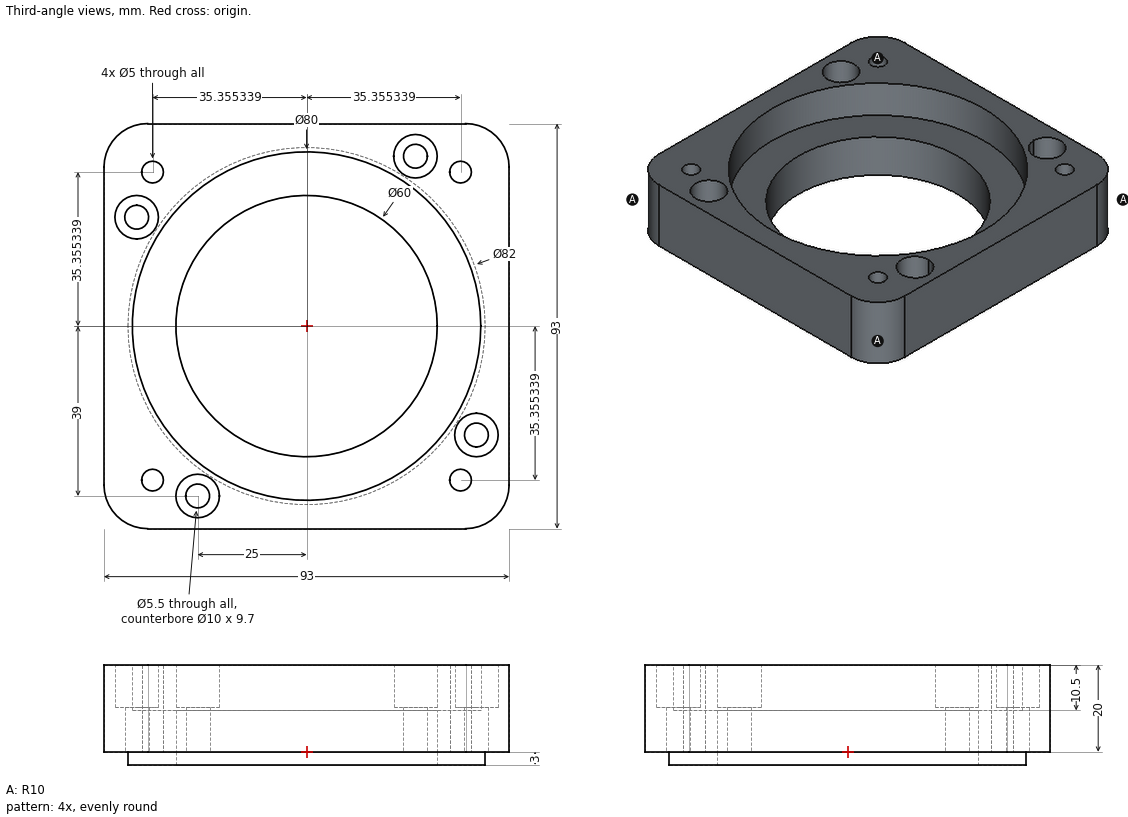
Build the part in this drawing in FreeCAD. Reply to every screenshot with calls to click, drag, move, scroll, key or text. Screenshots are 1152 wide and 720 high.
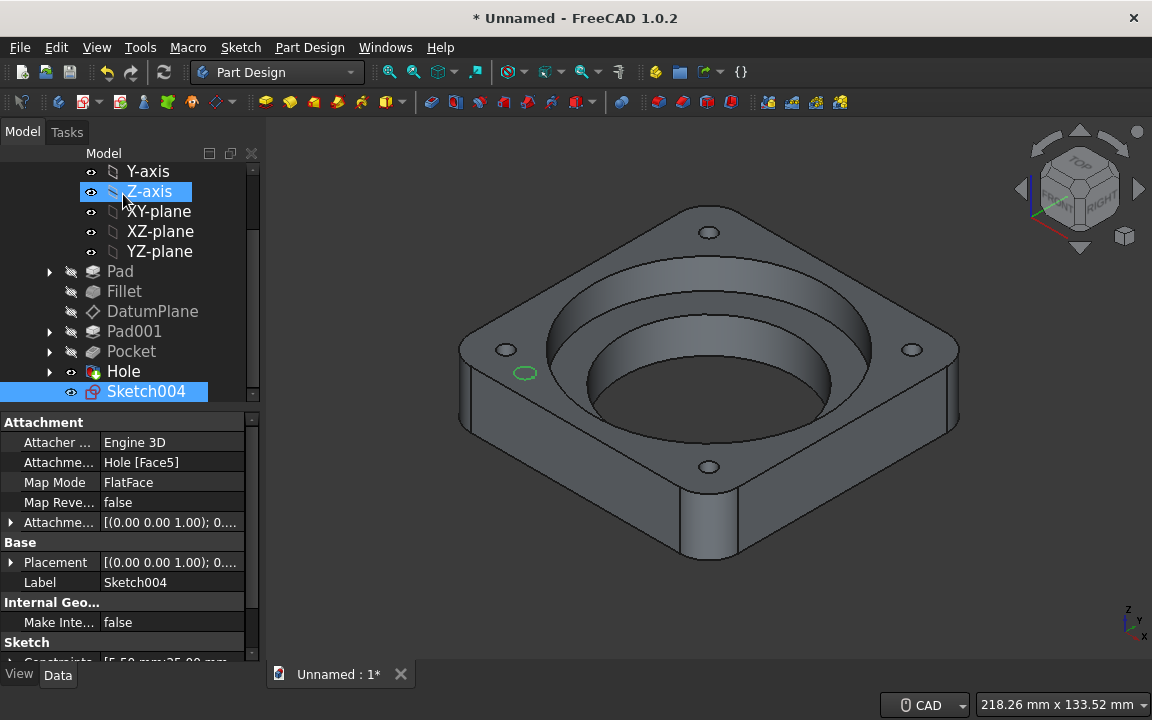
click(456, 102)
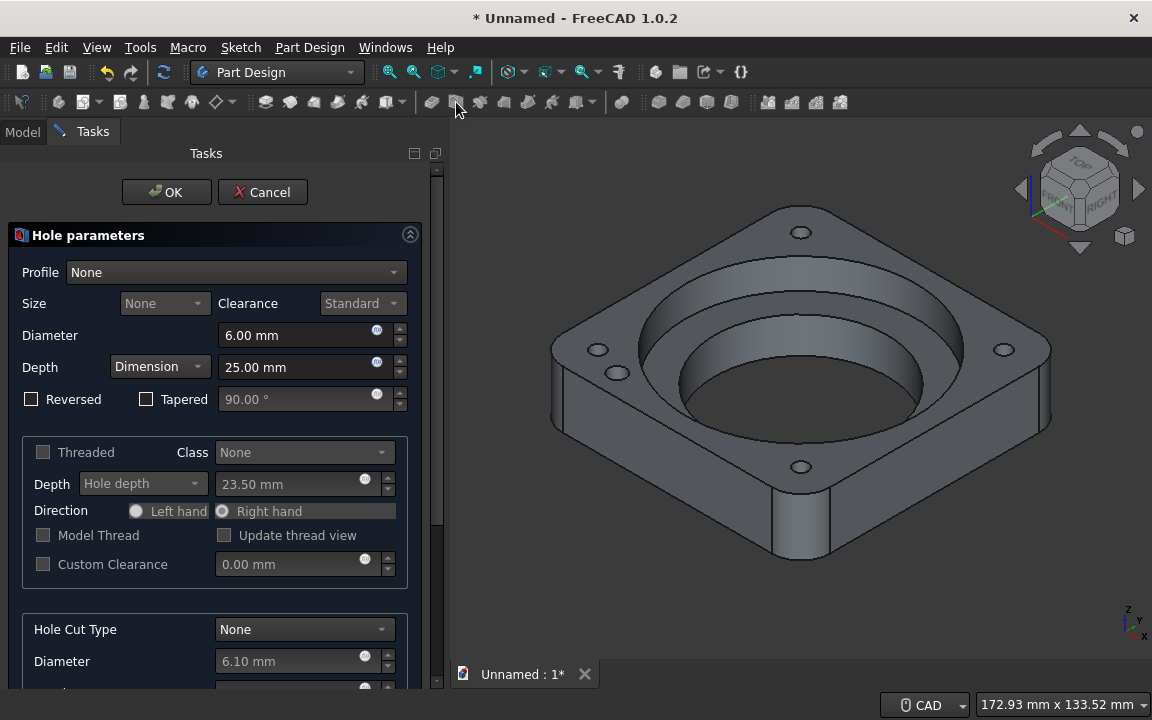
triple_click(305, 335)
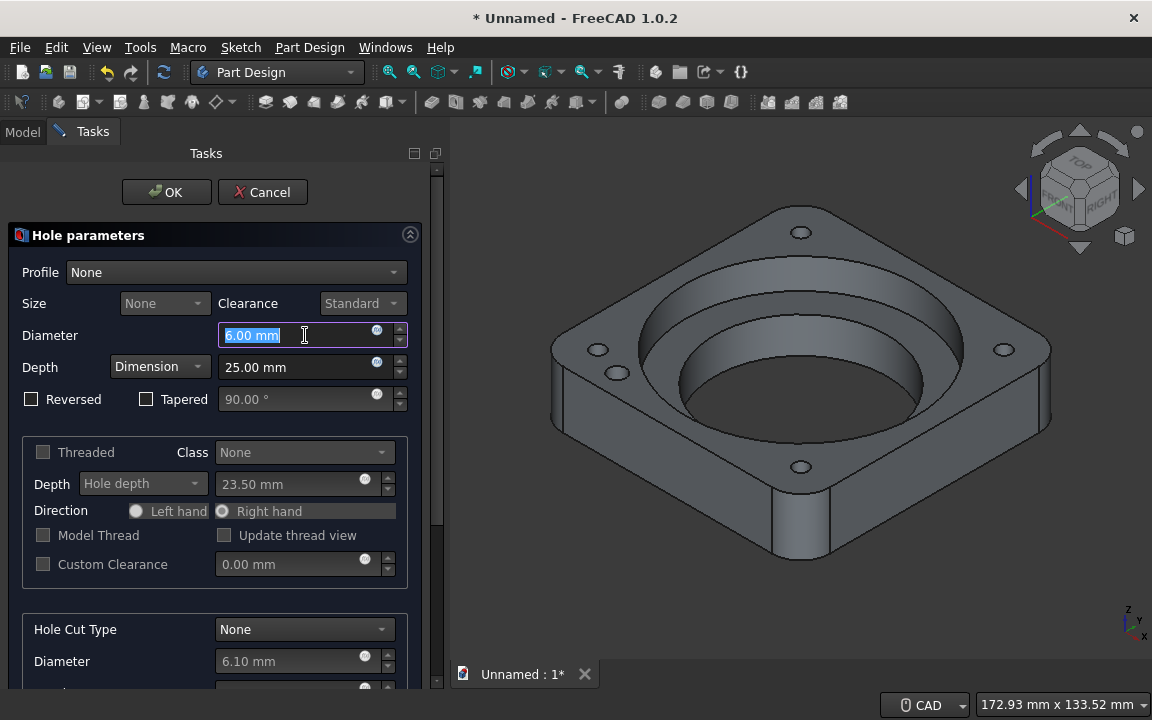
text(5.5)
key(Tab)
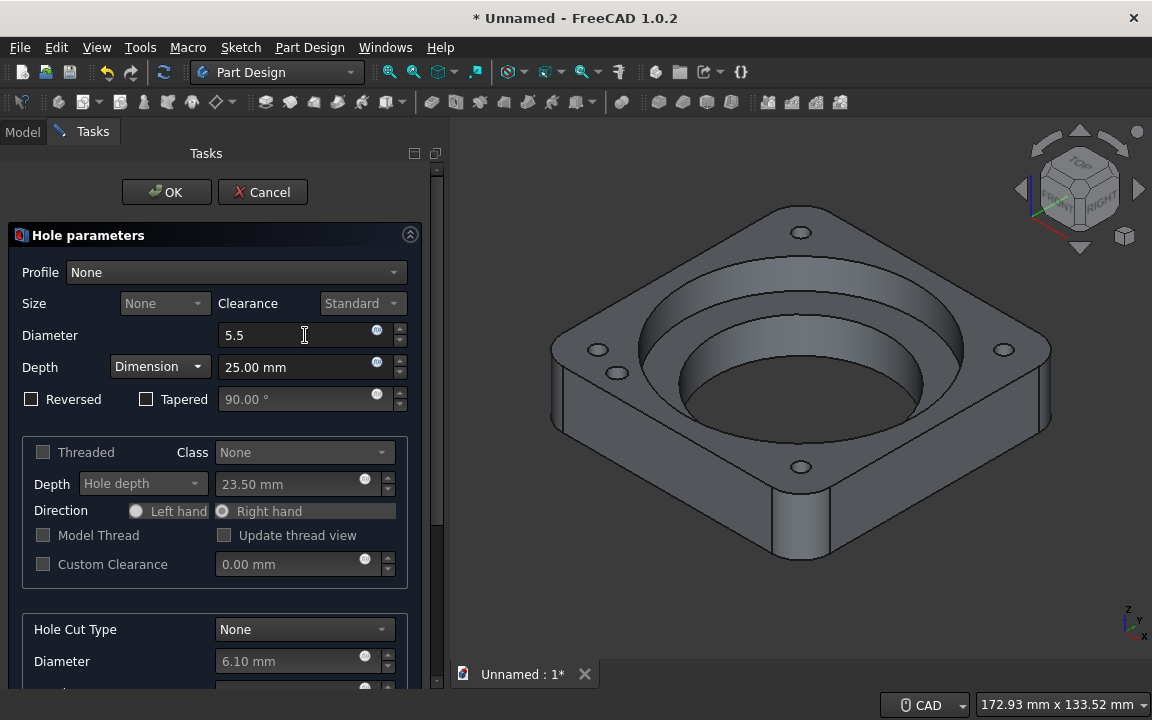
click(161, 366)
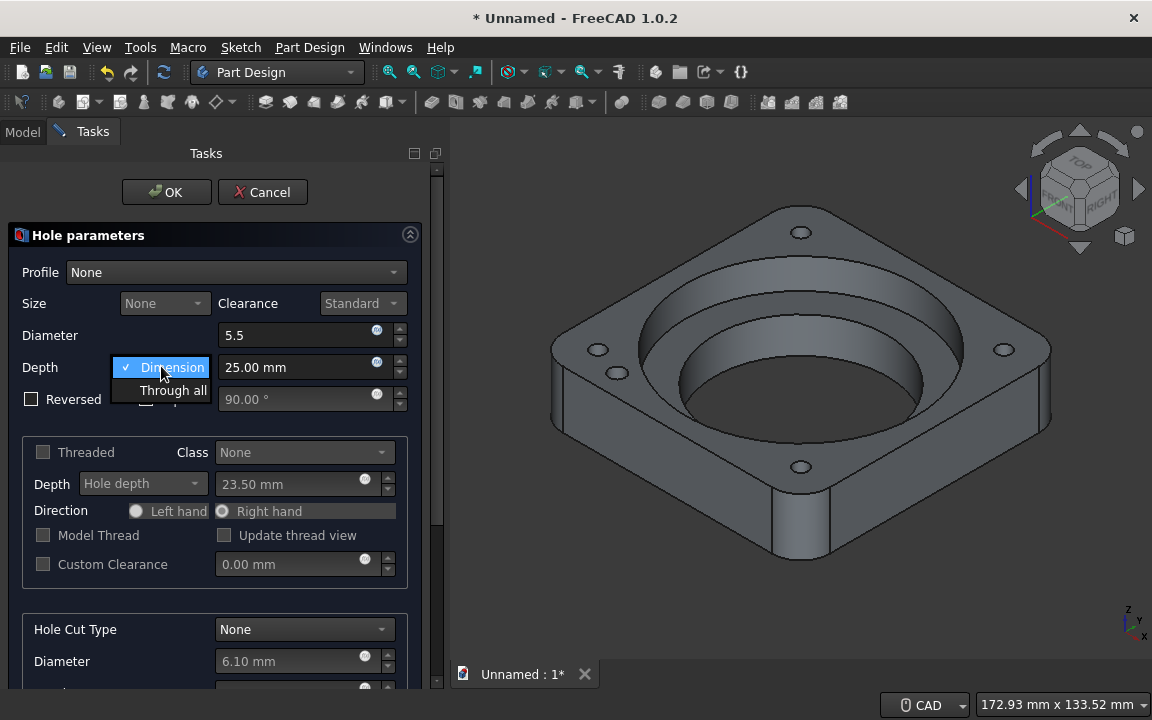
click(160, 390)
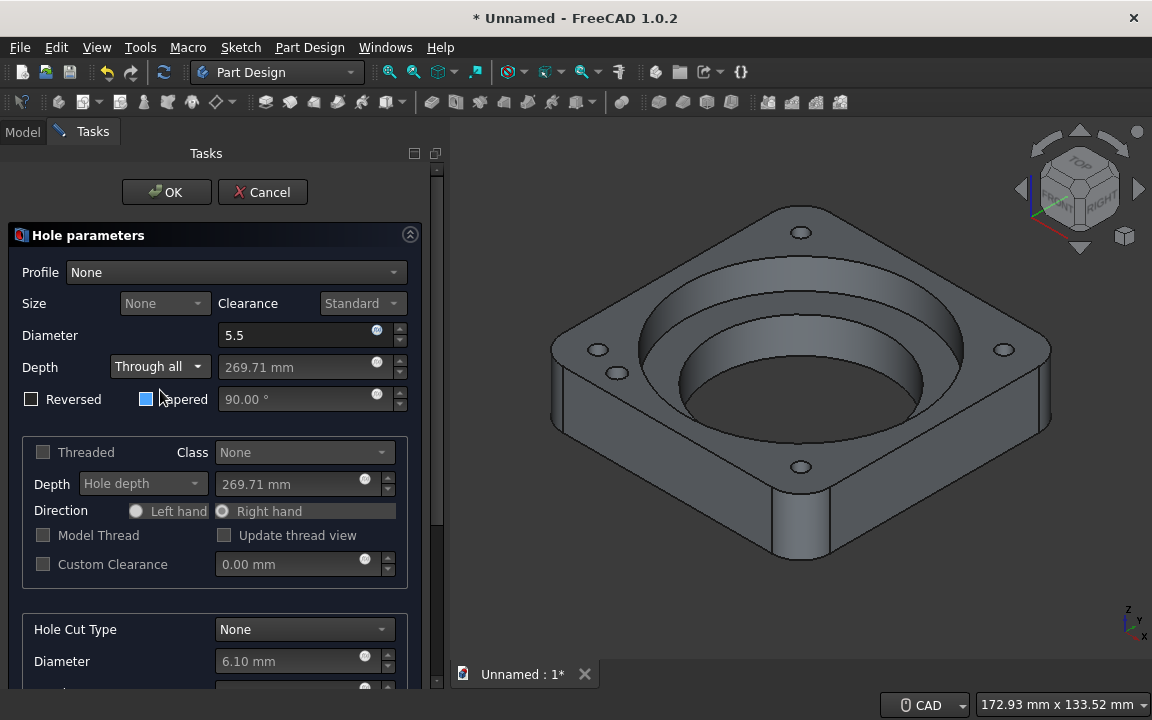
click(306, 630)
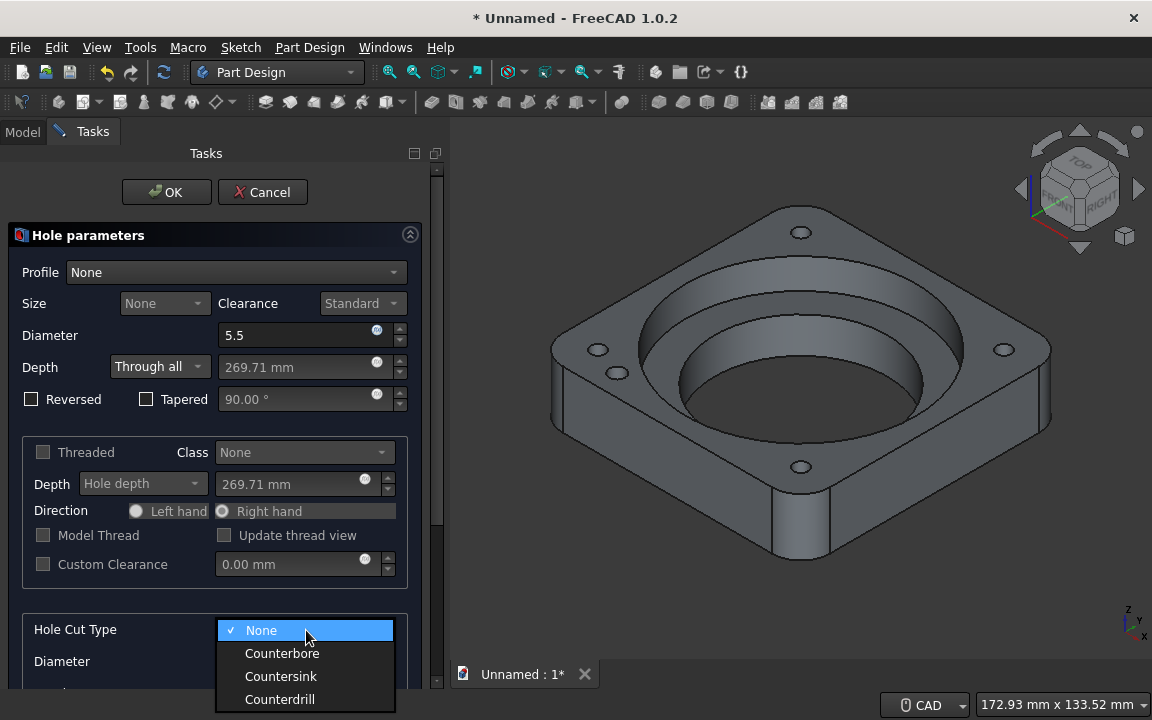
click(304, 654)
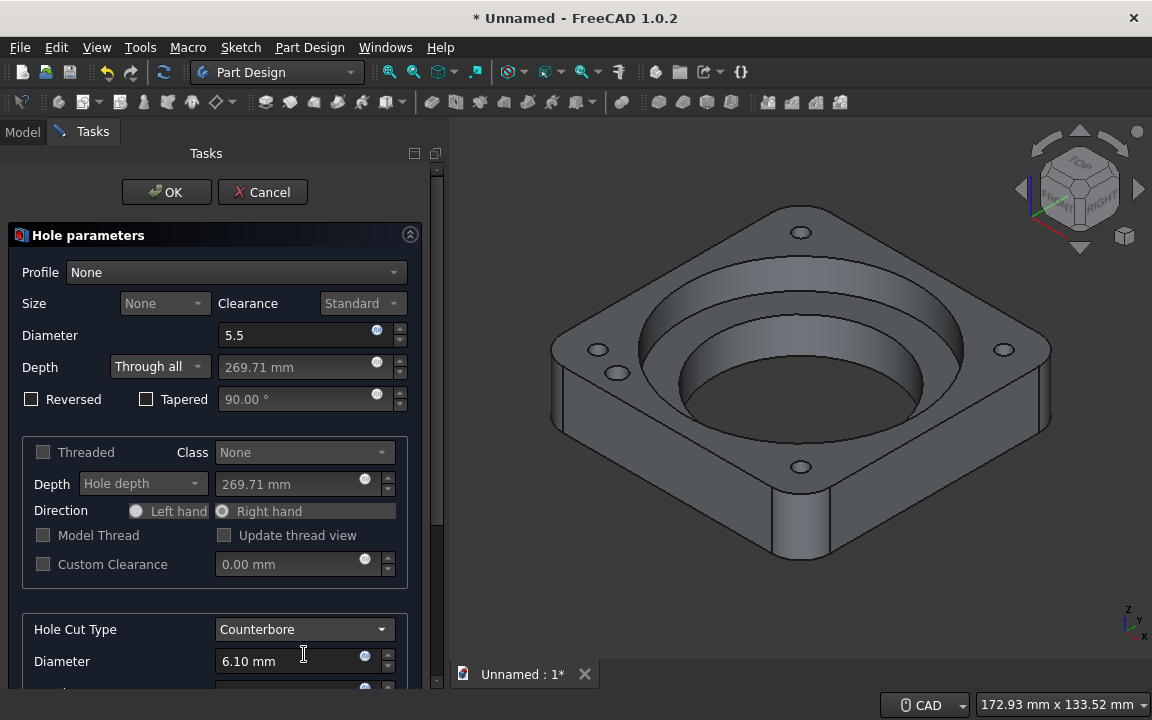
triple_click(298, 661)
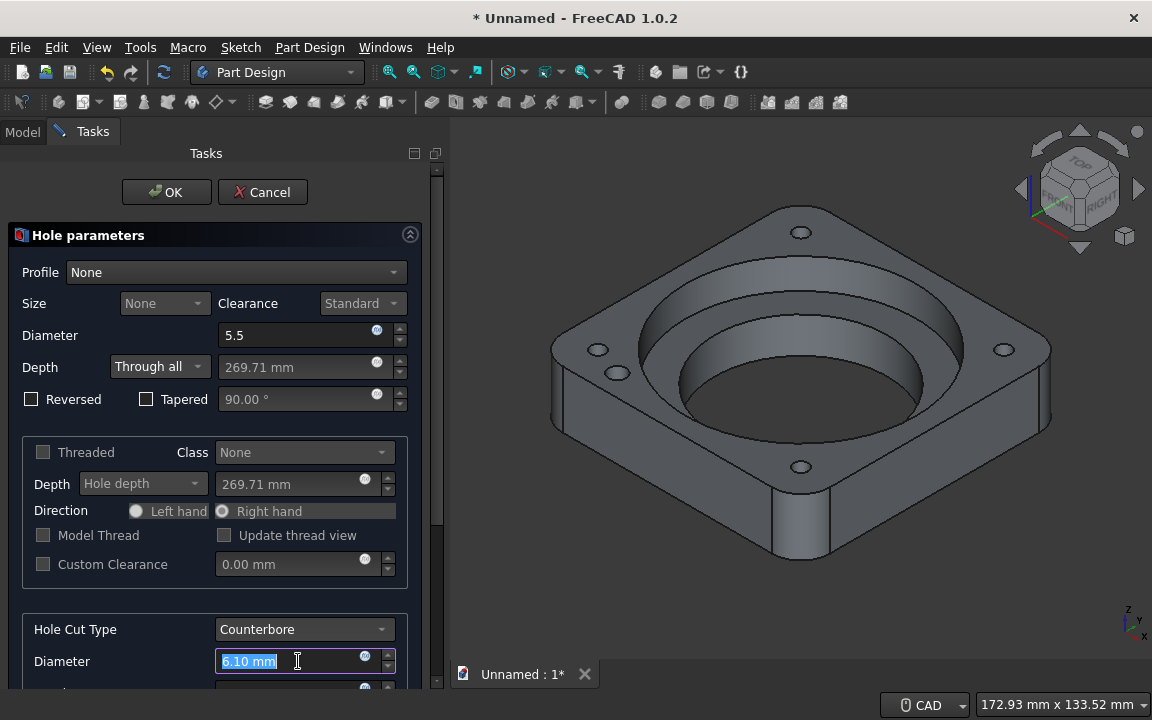
text(10)
key(Tab)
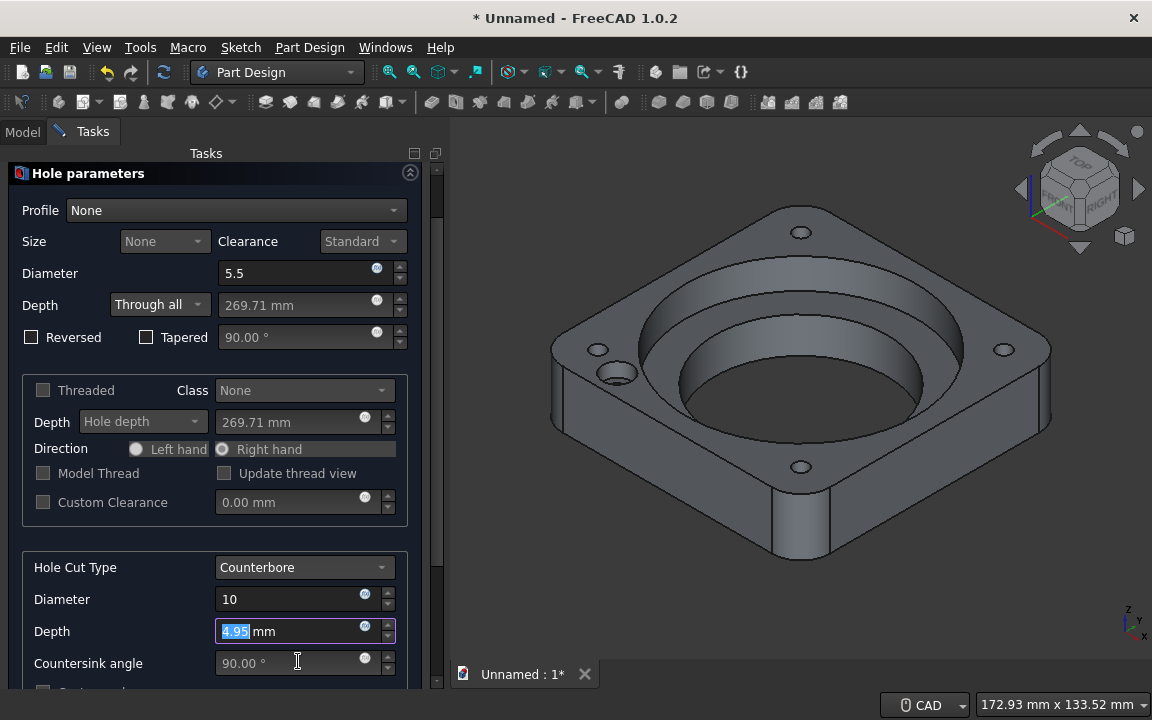
text(9.7)
key(Tab)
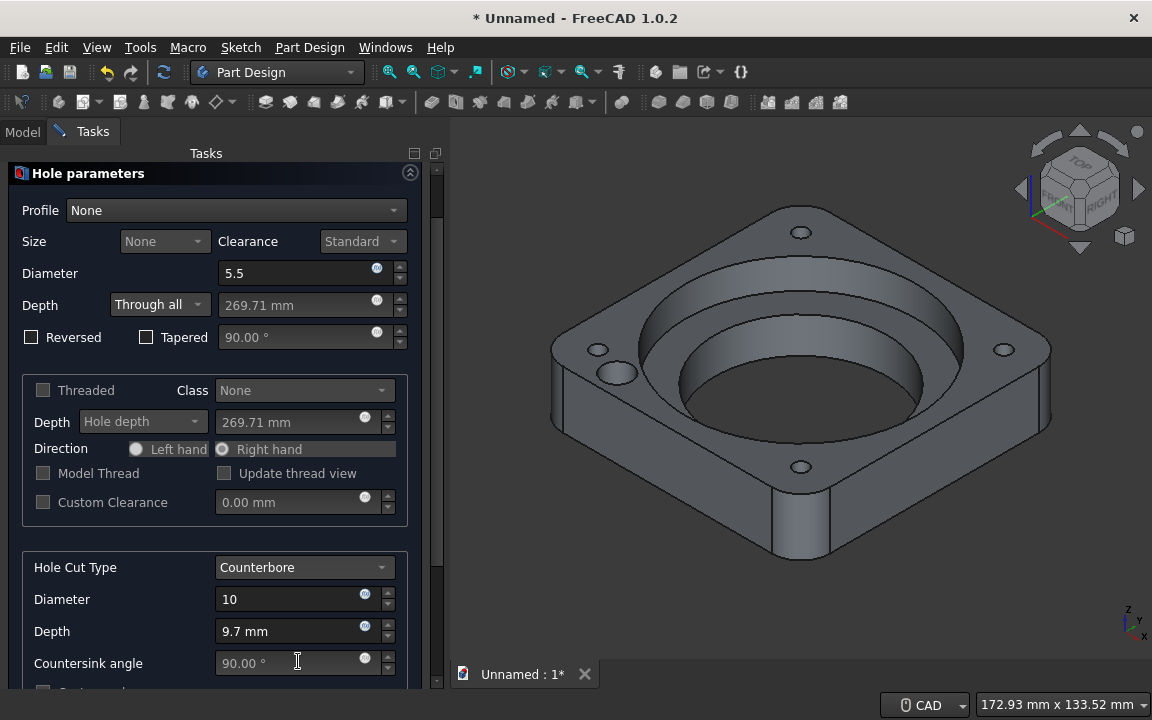
scroll(437, 426, up, 2)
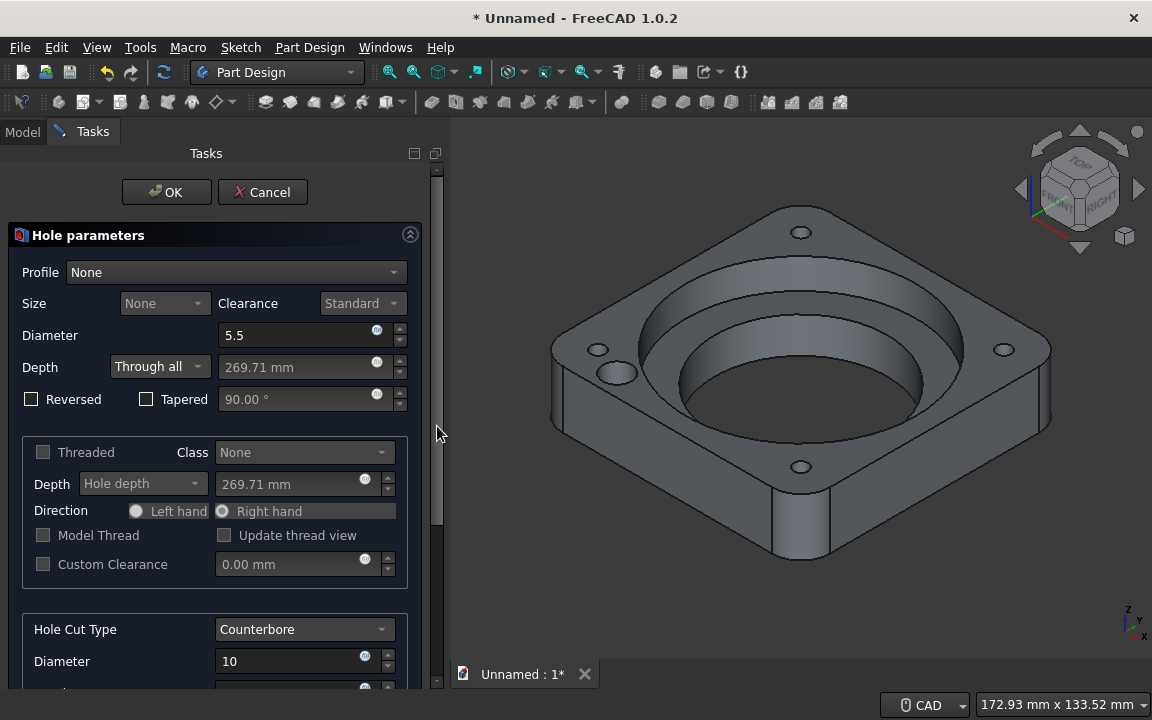
click(167, 192)